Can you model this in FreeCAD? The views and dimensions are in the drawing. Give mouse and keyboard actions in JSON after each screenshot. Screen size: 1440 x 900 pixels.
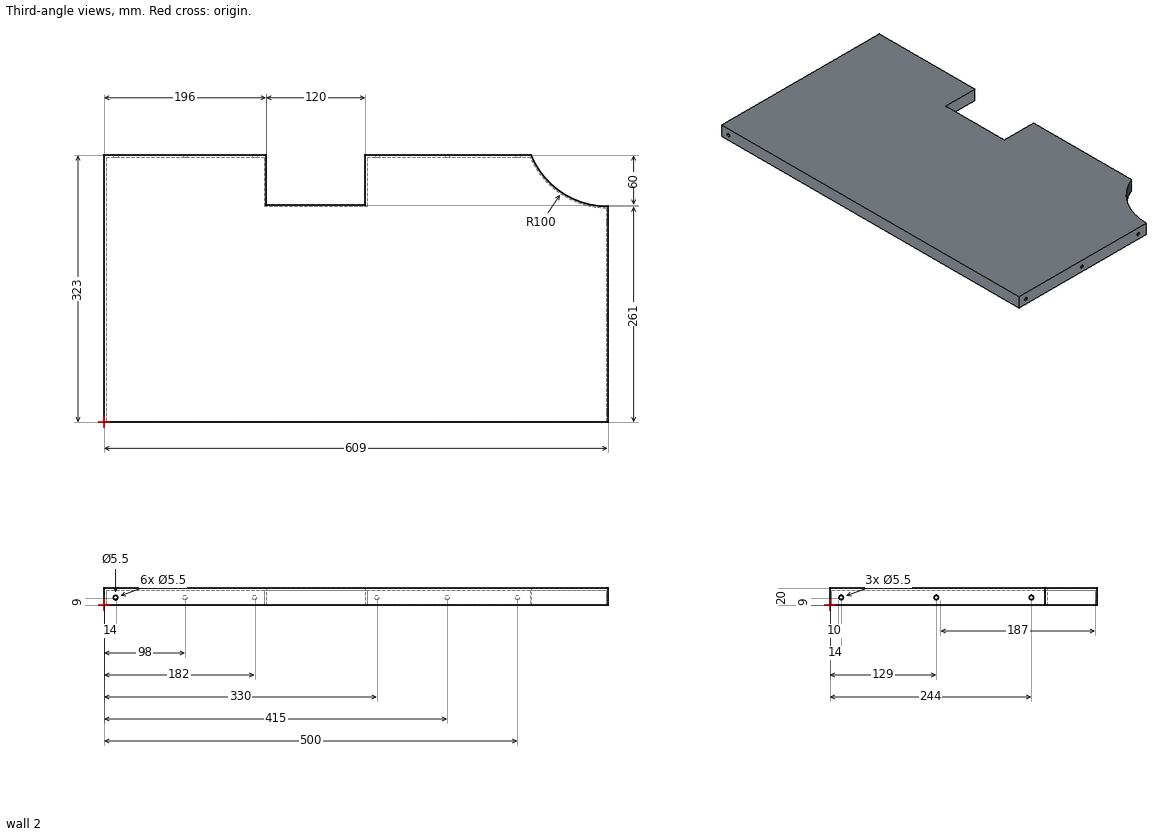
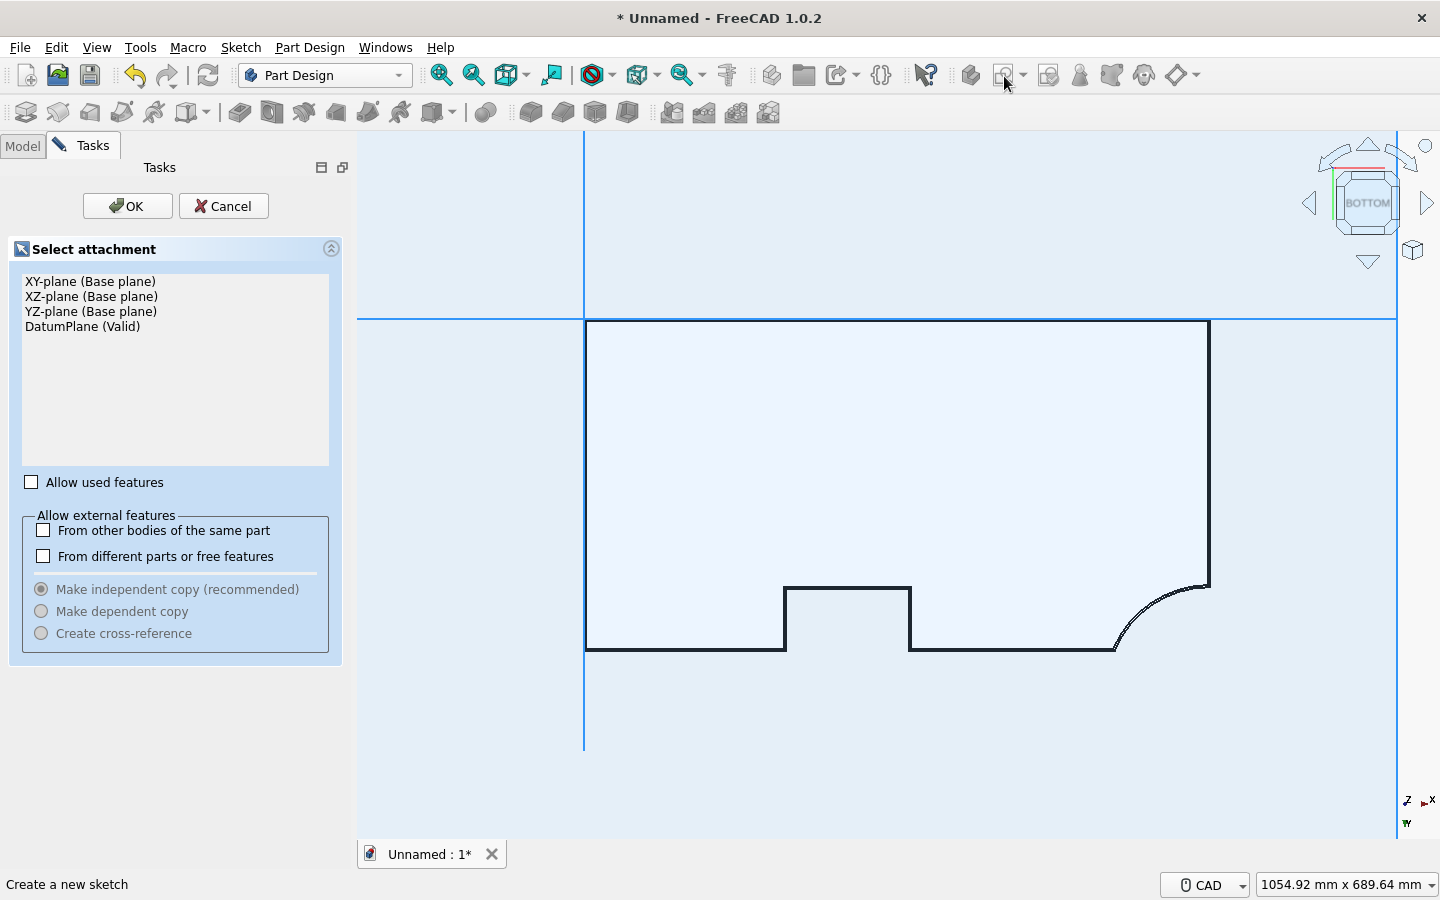
{"action": "left_click", "coordinate": [82, 296]}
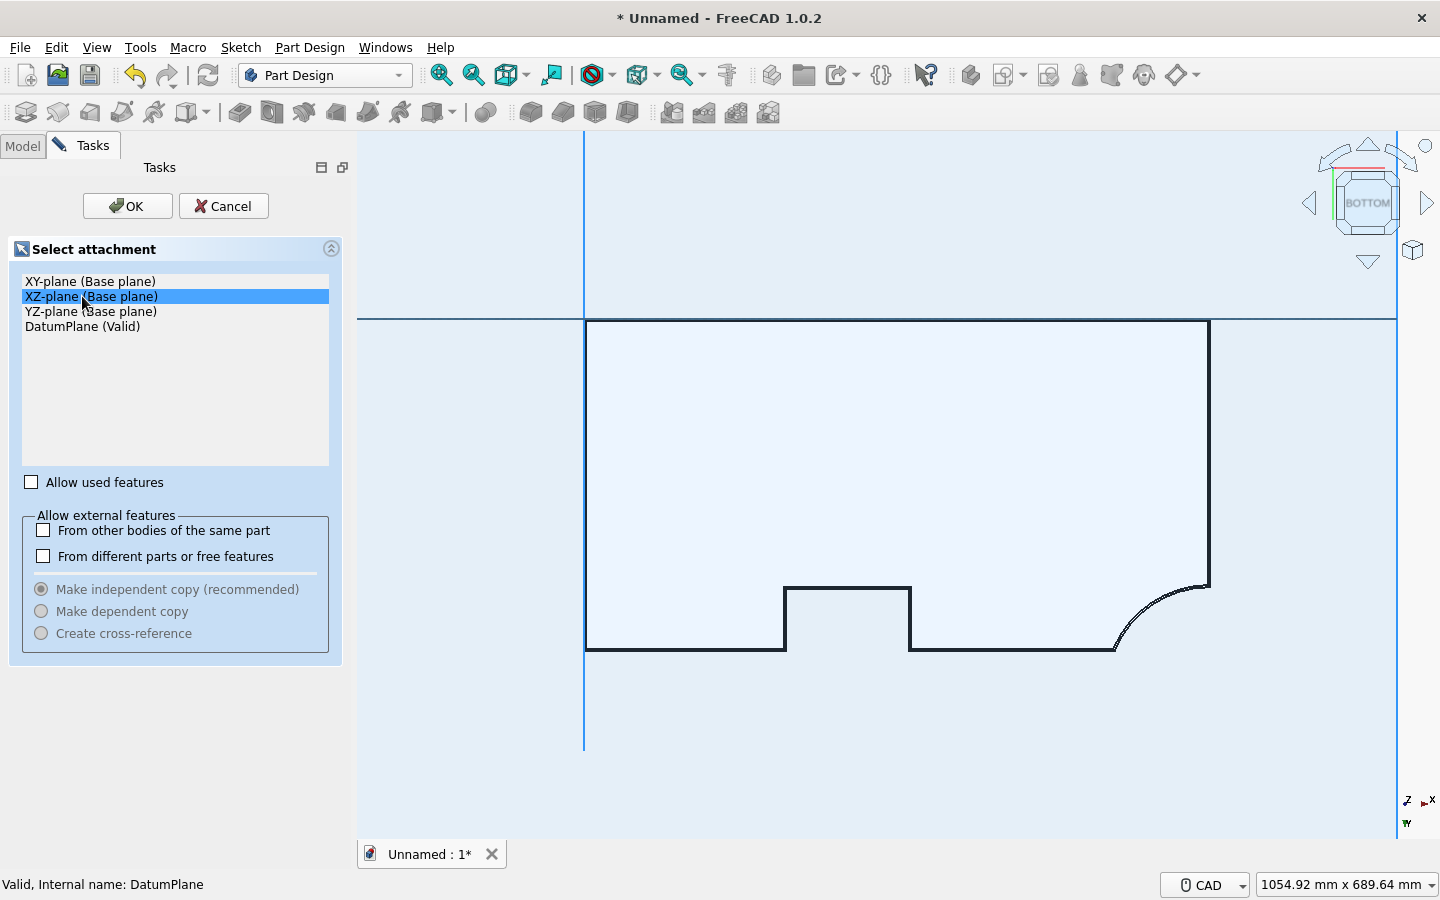
{"action": "left_click", "coordinate": [128, 206]}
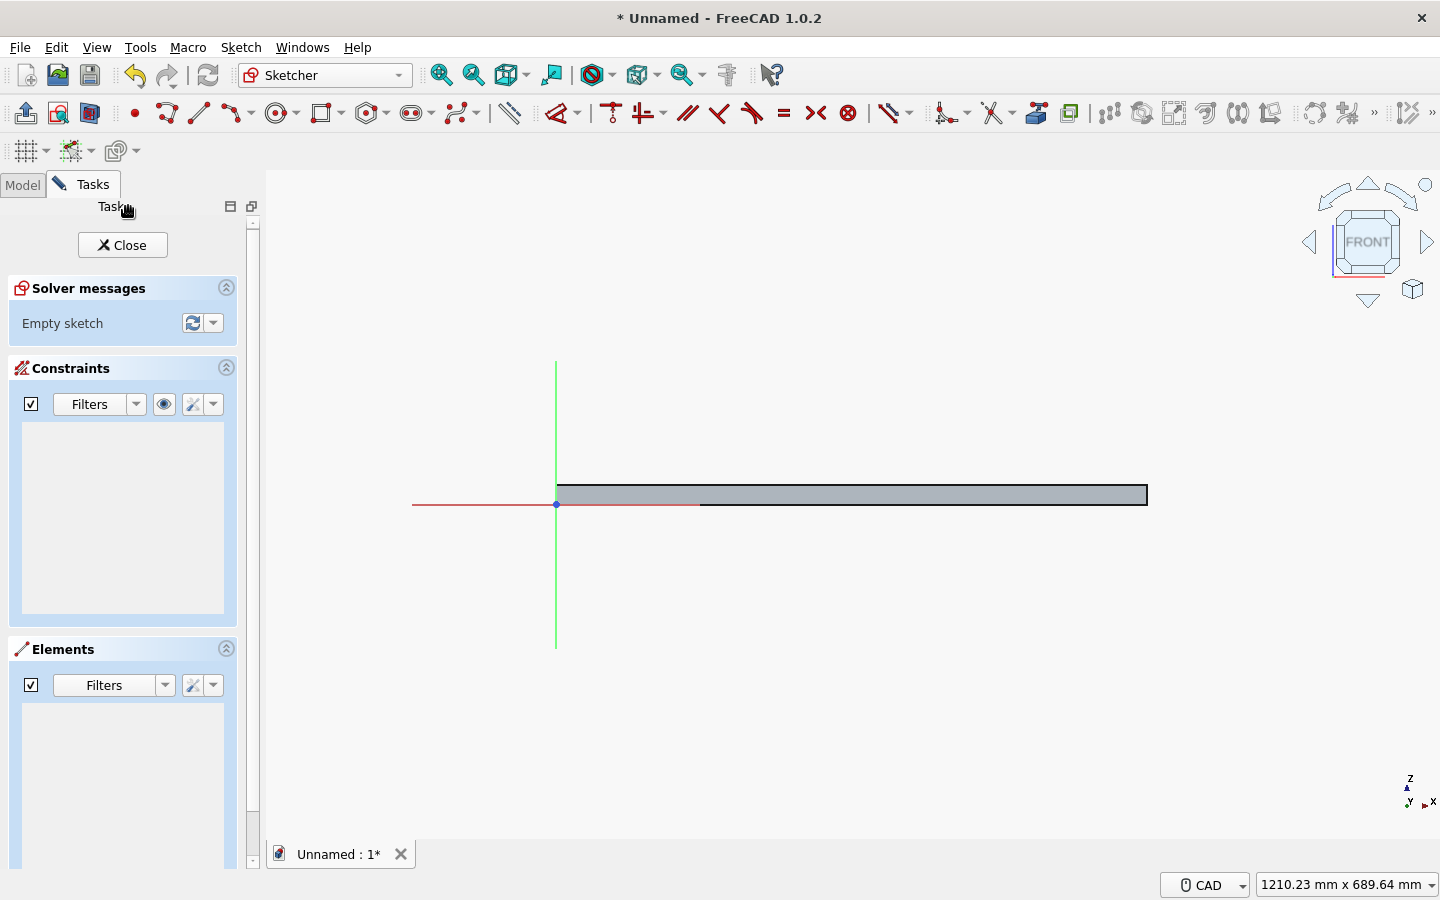
{"action": "scroll", "coordinate": [559, 496], "scroll_direction": "up", "scroll_amount": 15}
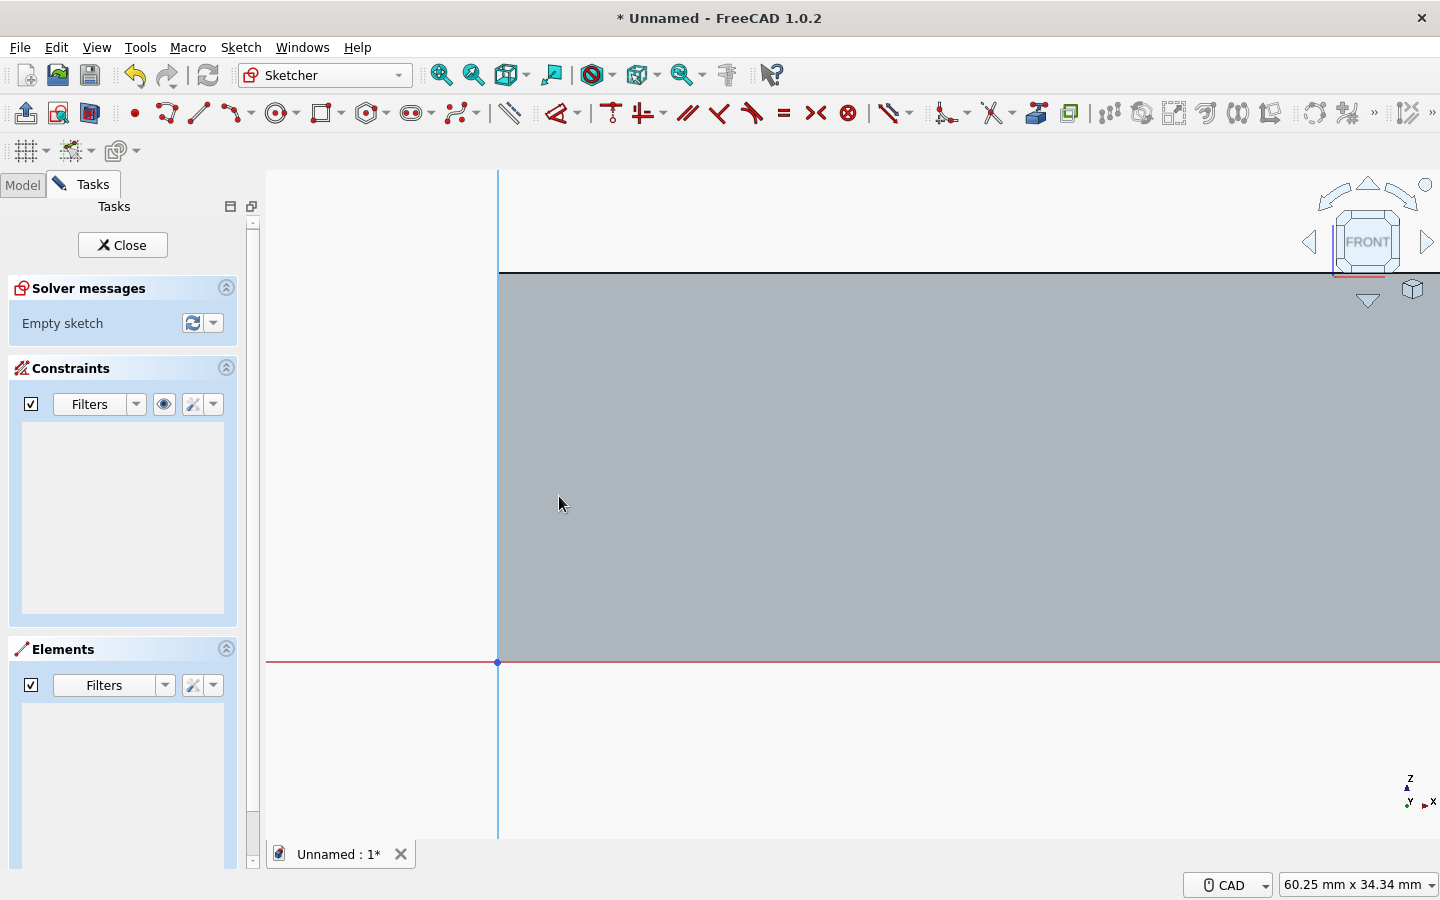
{"action": "scroll", "coordinate": [766, 481], "scroll_direction": "up", "scroll_amount": 7}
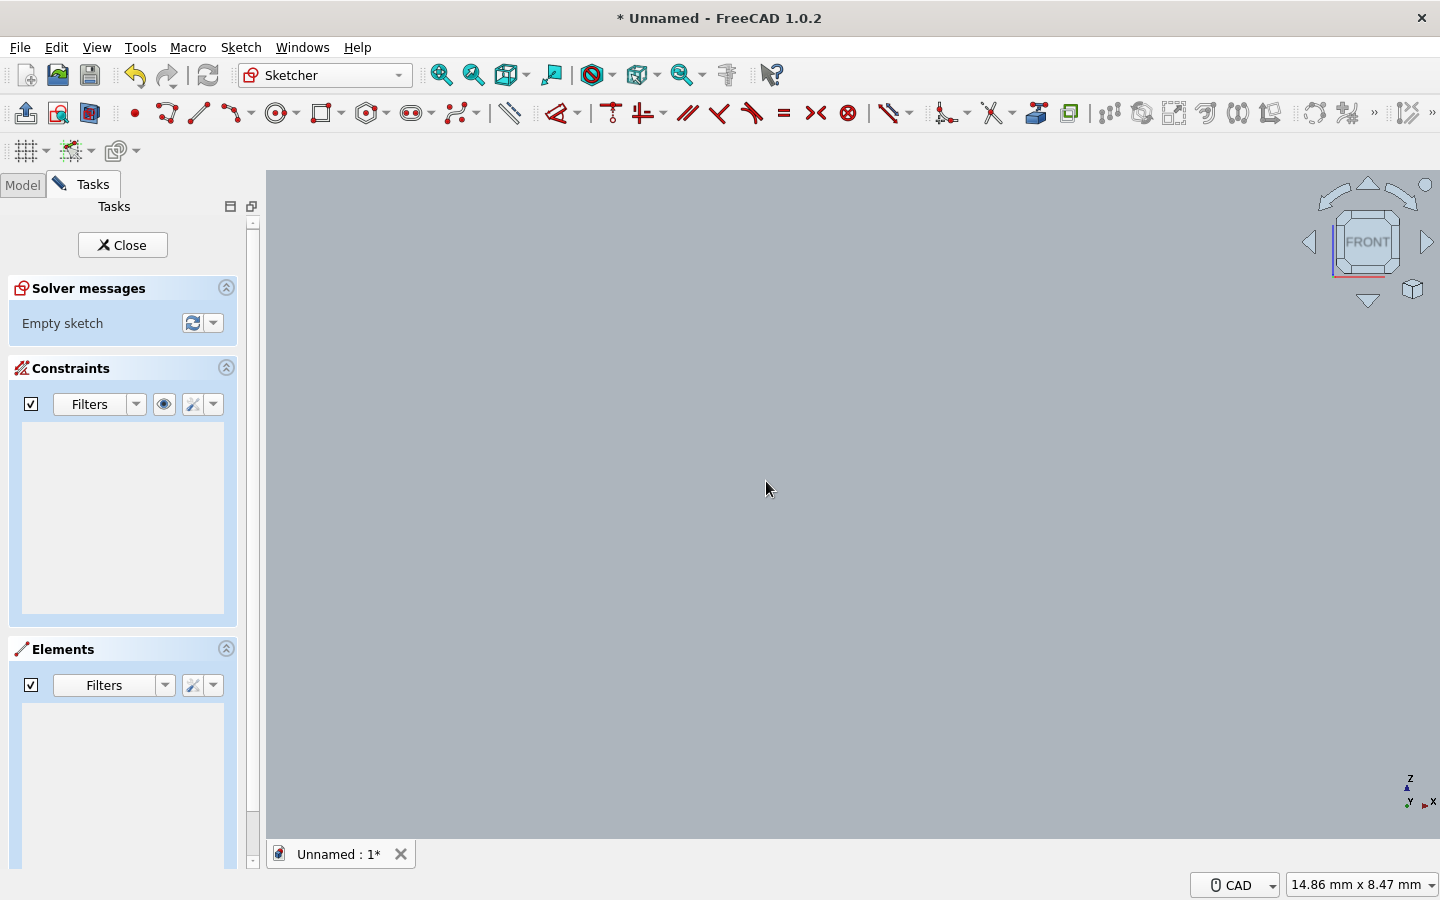
{"action": "left_click", "coordinate": [276, 114]}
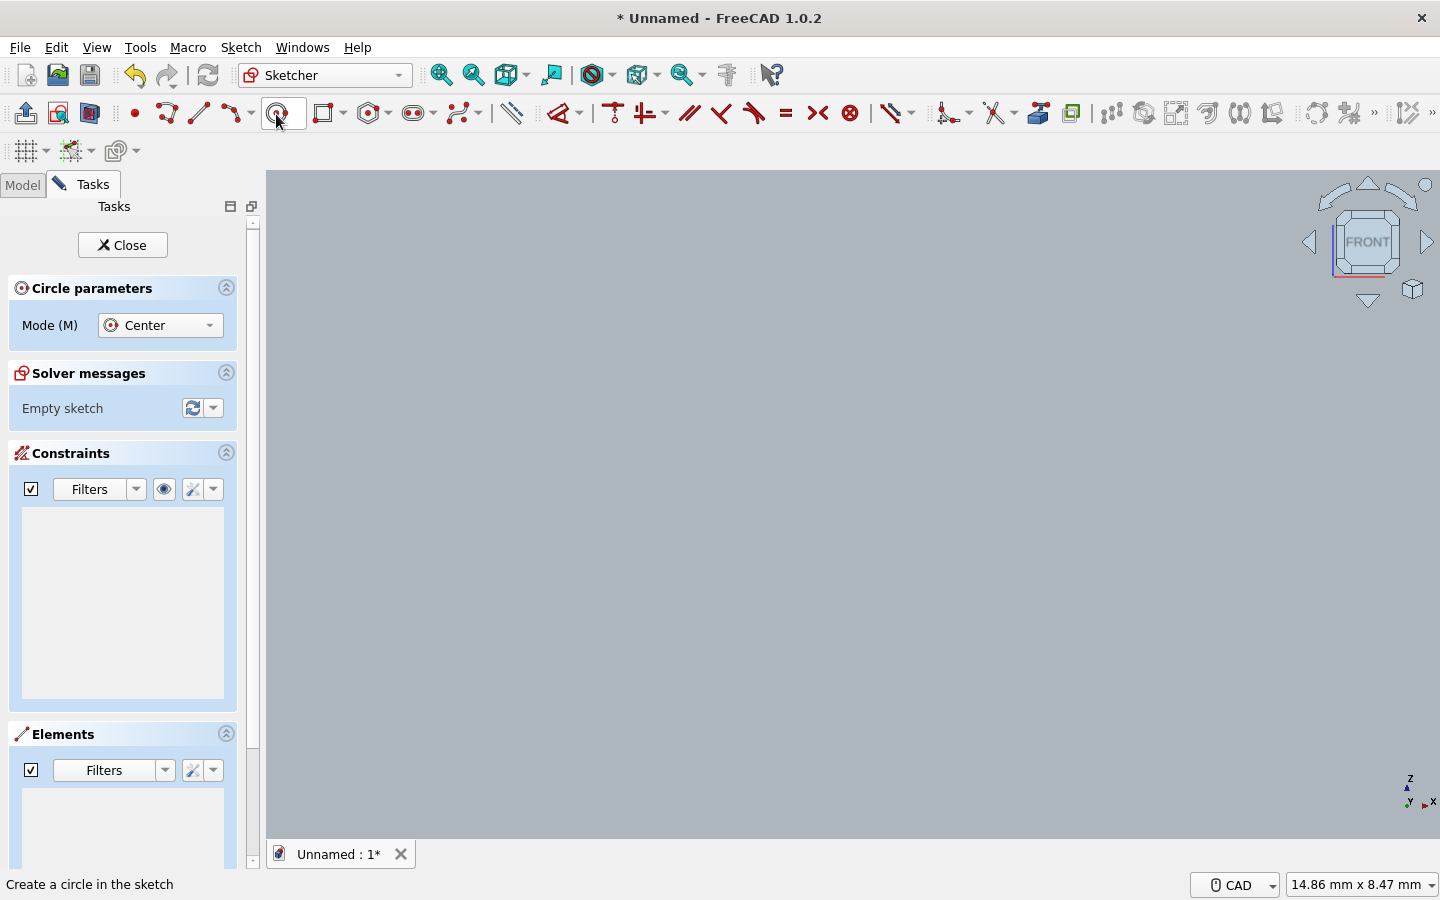
{"action": "left_click", "coordinate": [784, 504]}
{"action": "mouse_move", "coordinate": [938, 351]}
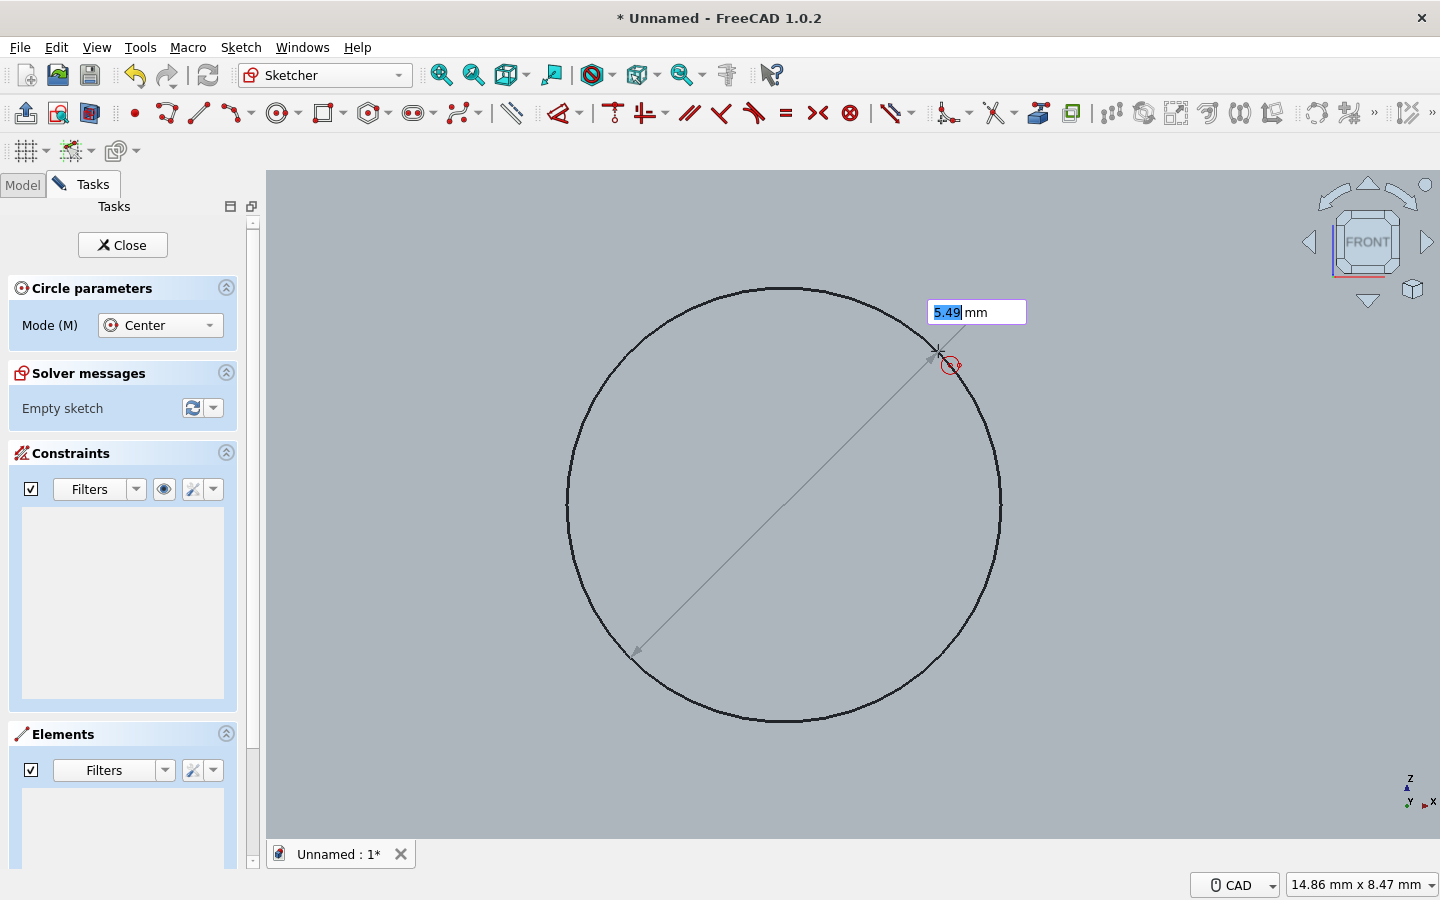
{"action": "type", "text": "5.5"}
{"action": "key", "text": "Return"}
{"action": "key", "text": "Escape"}